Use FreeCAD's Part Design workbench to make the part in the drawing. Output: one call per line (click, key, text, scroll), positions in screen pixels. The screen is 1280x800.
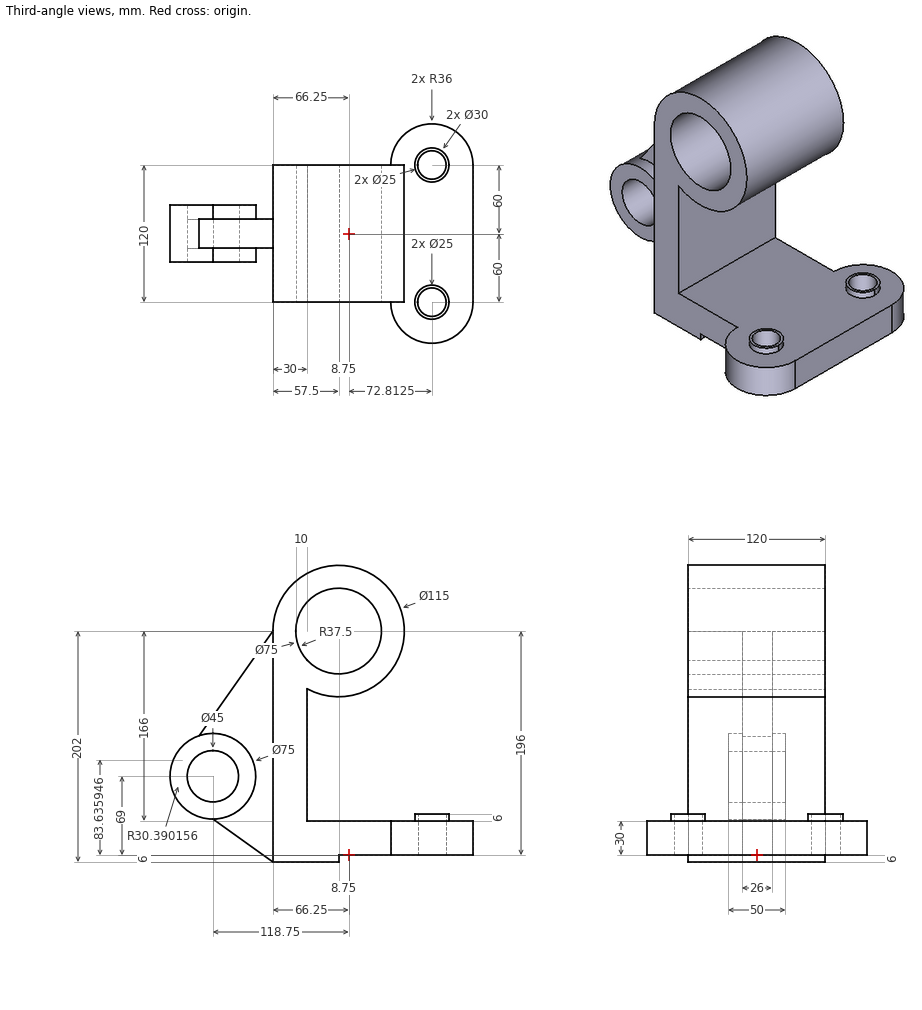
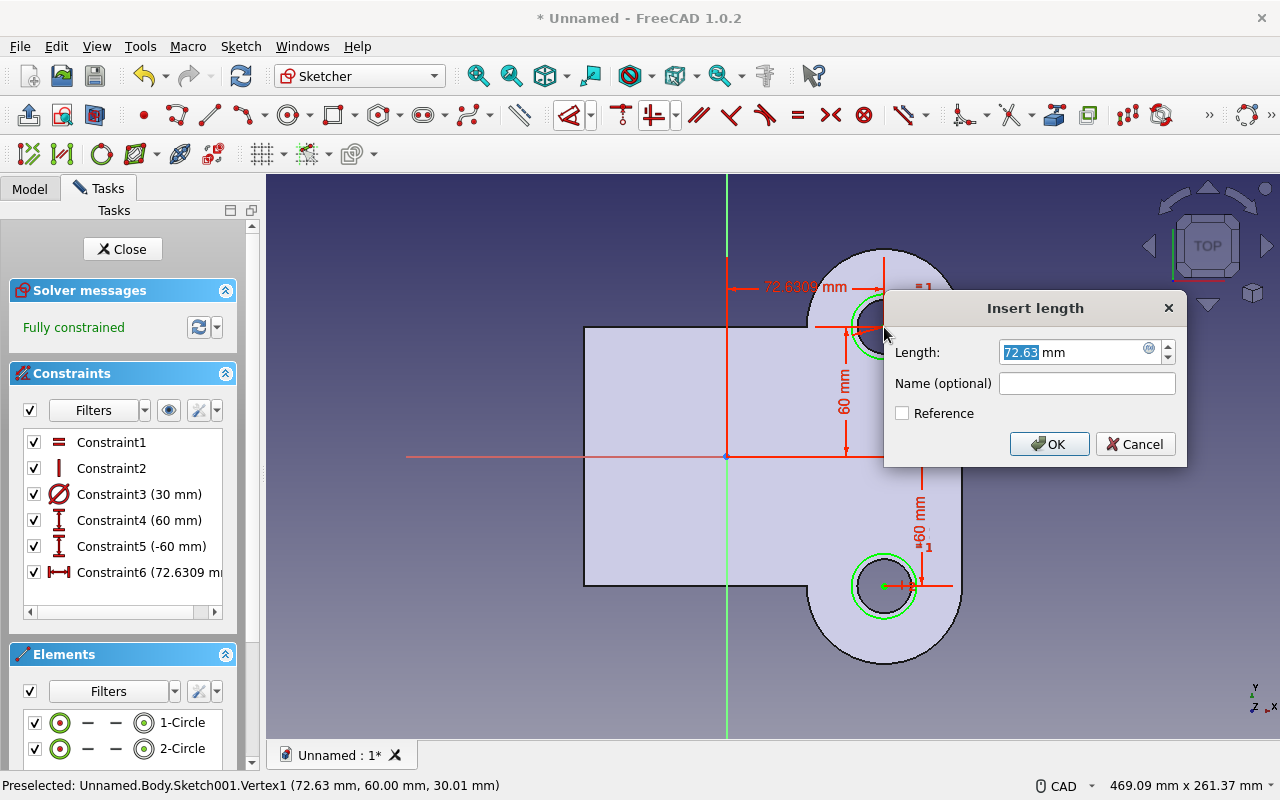
text(72.8125)
key(Return)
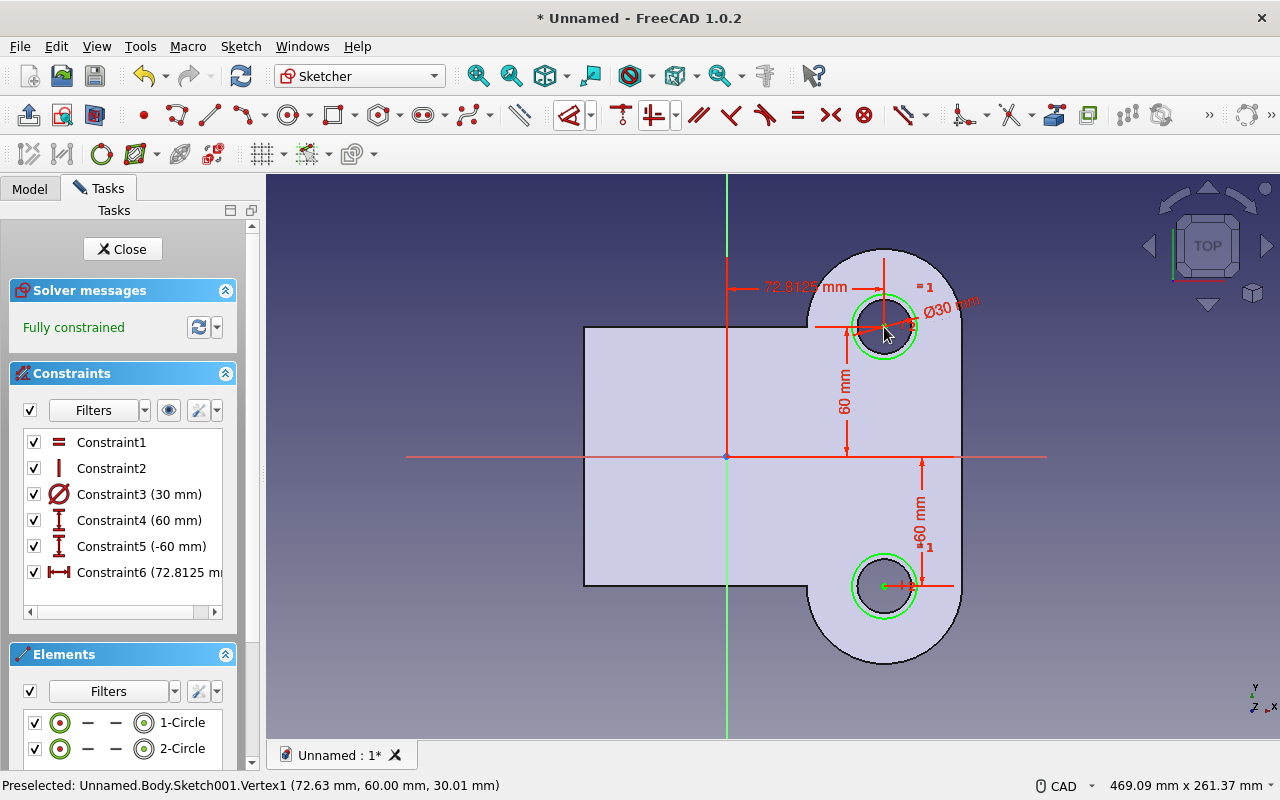
click(123, 249)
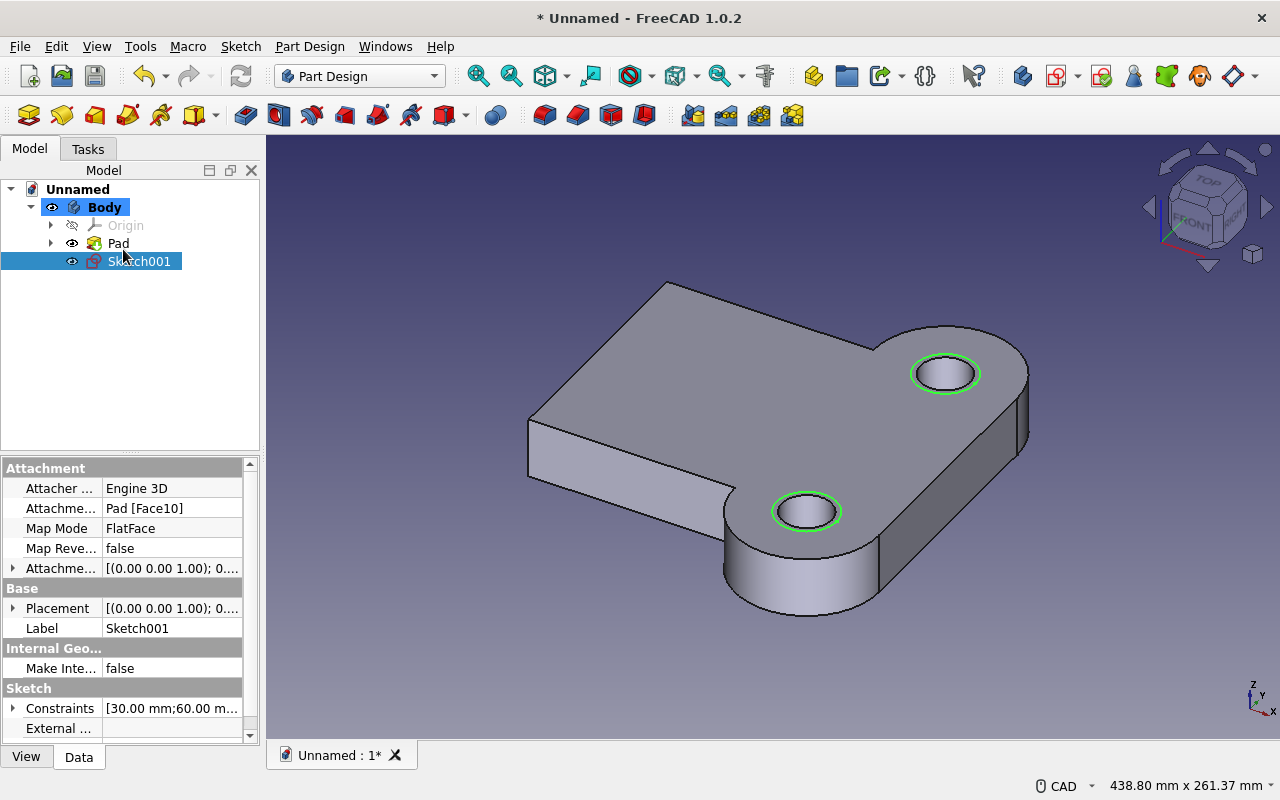
click(29, 116)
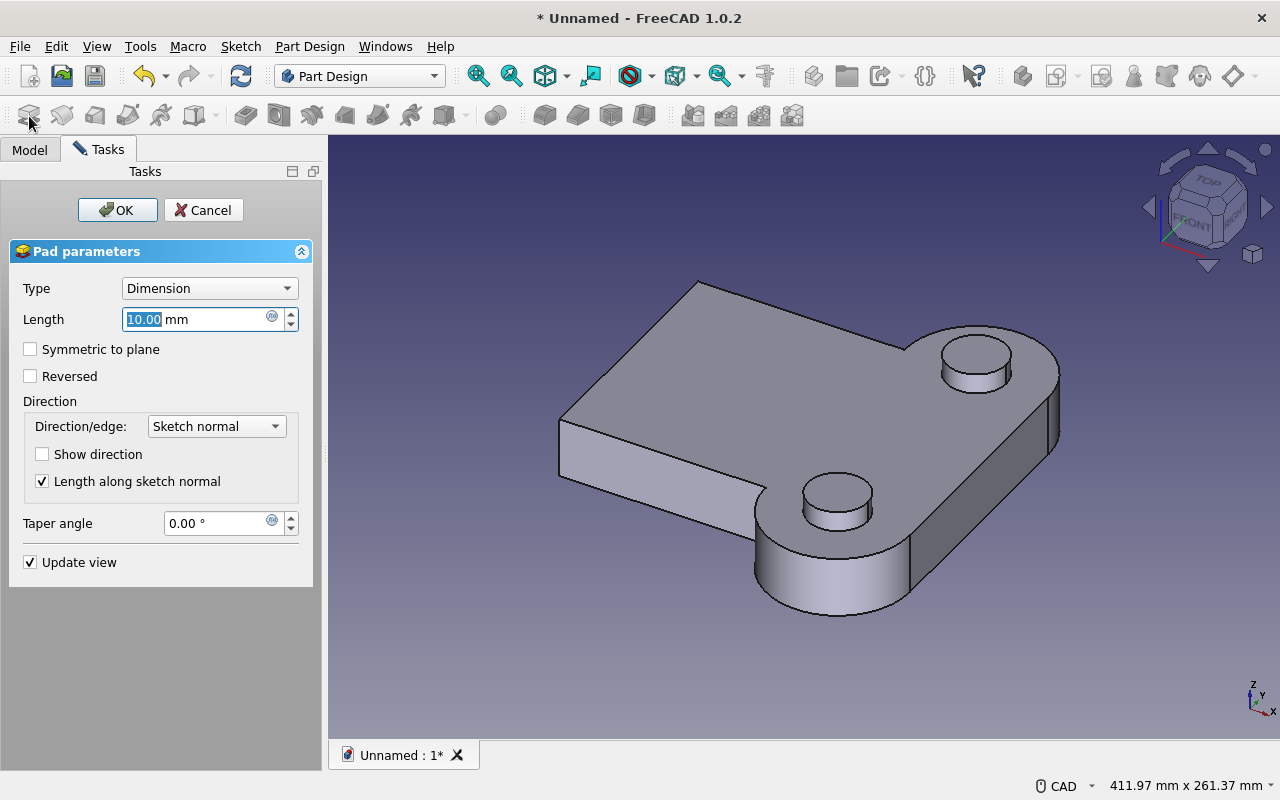
text(6)
key(Tab)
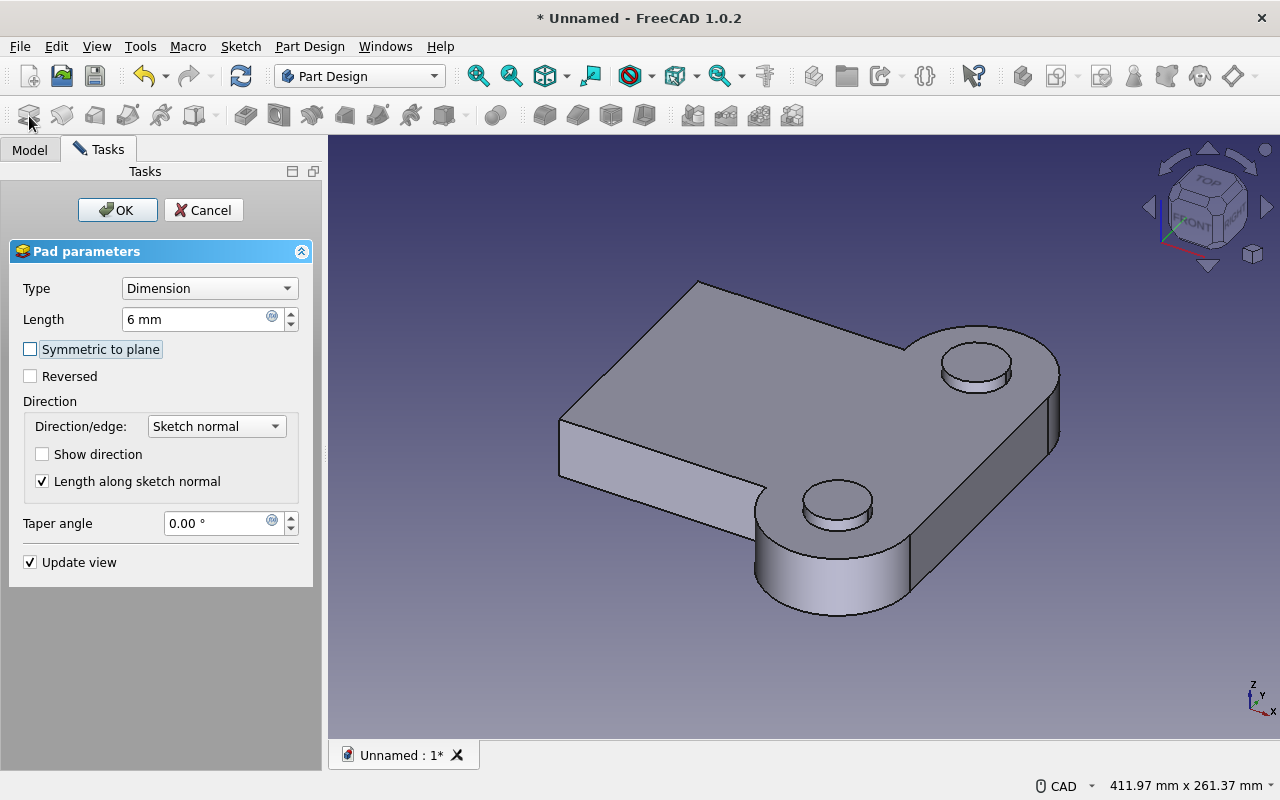
click(118, 210)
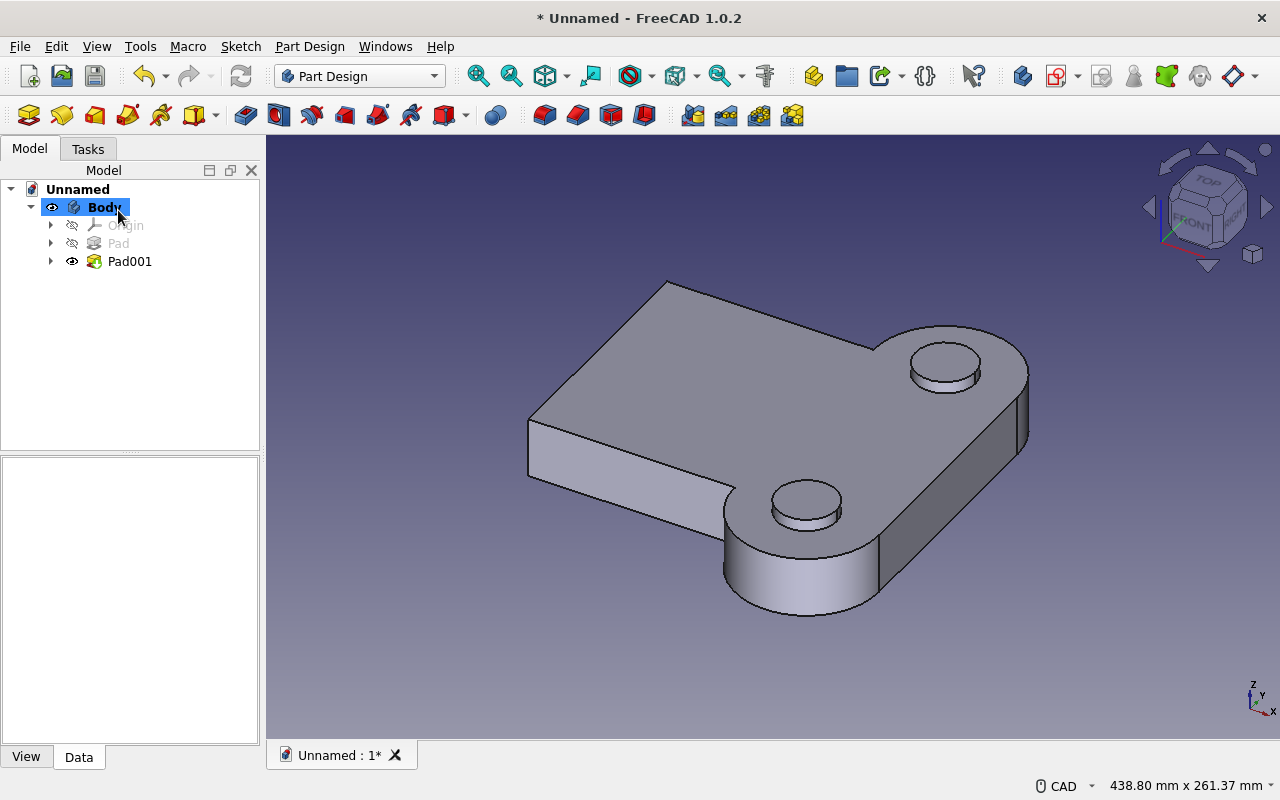
key(5)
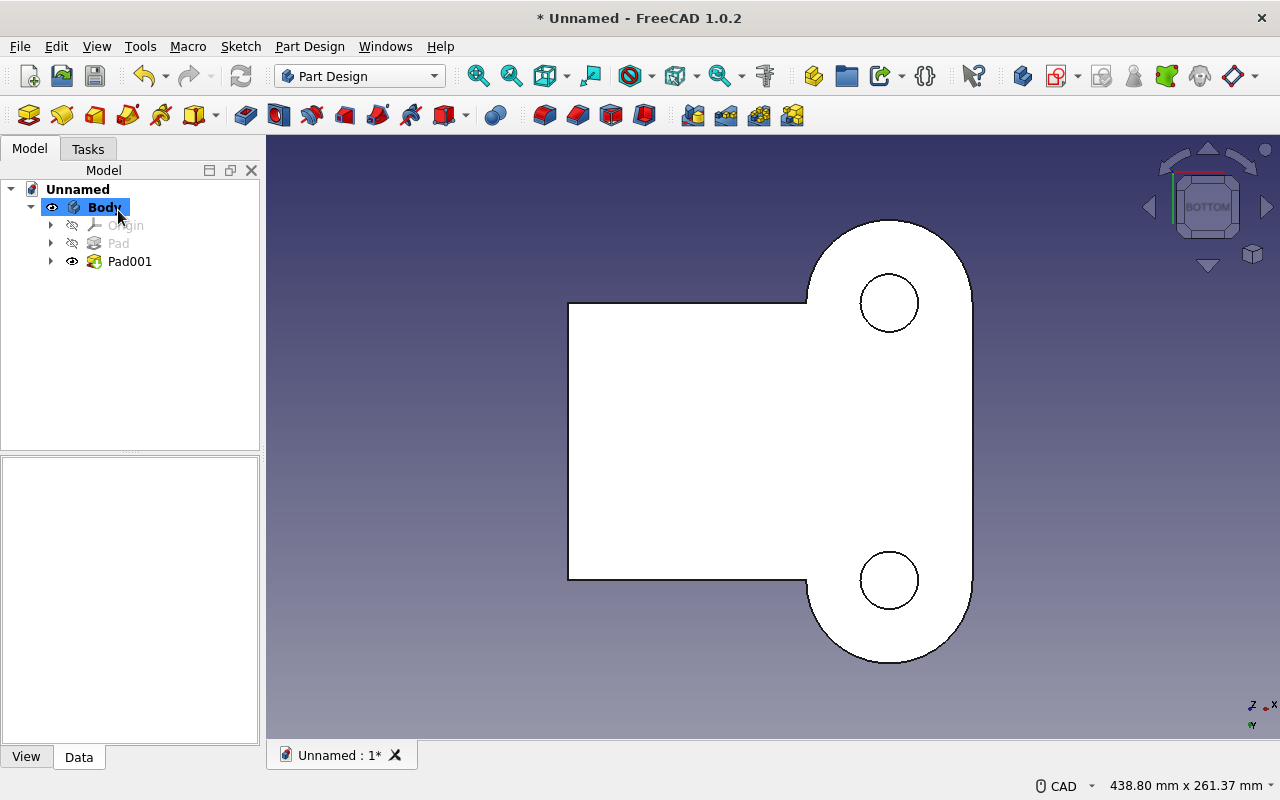
click(770, 441)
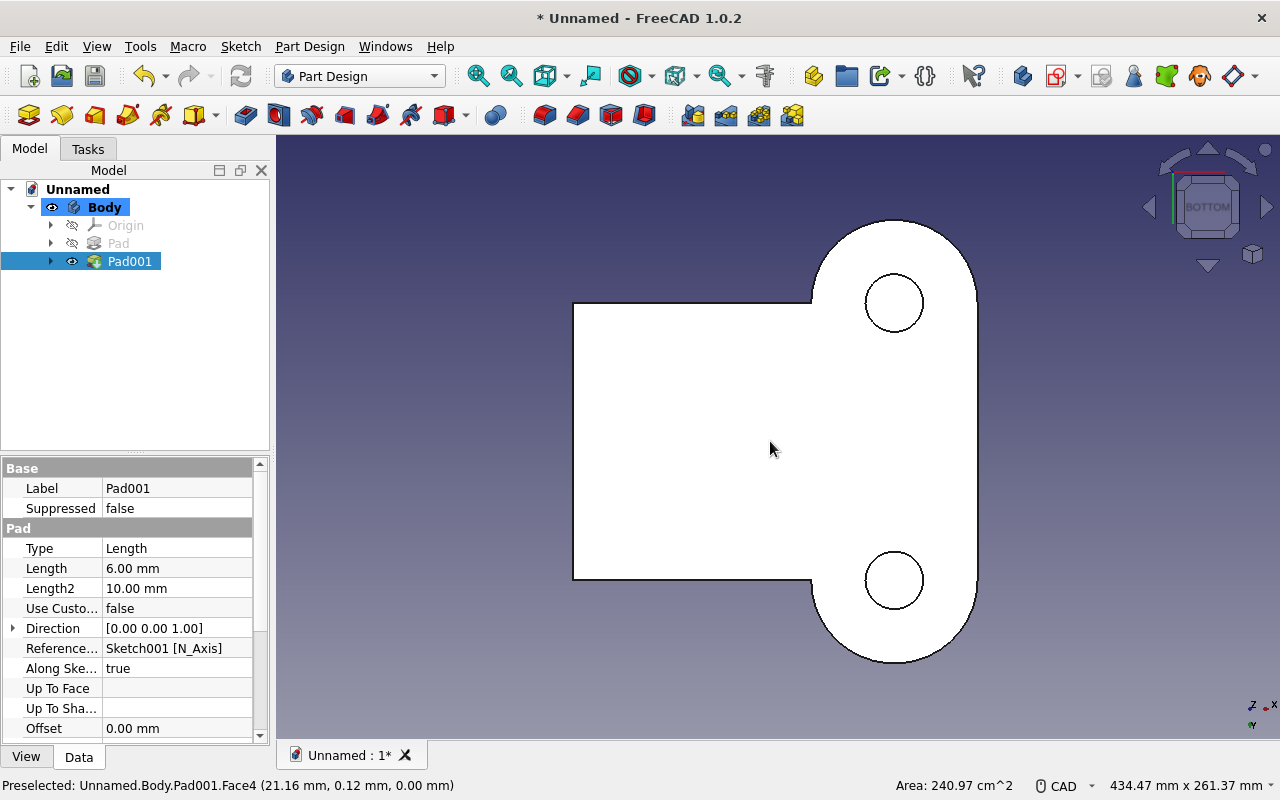
click(1056, 76)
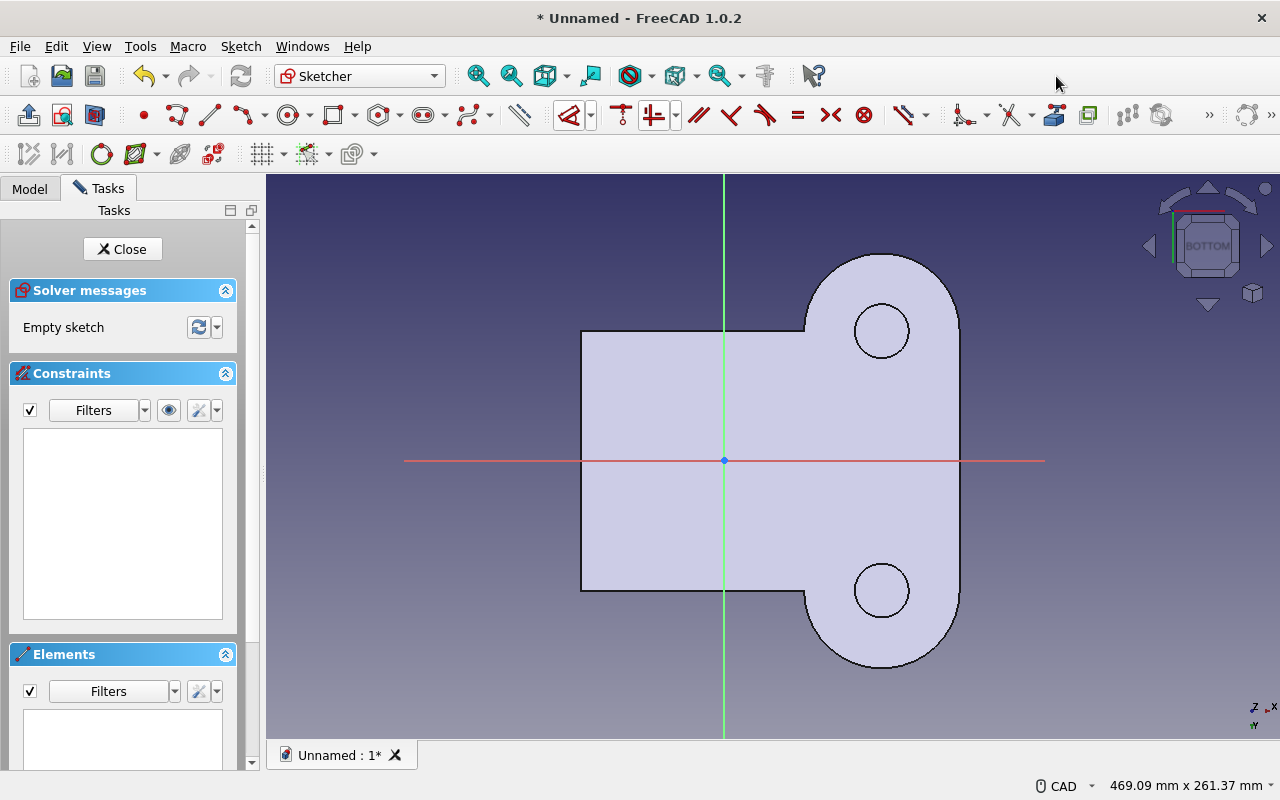
key(g)
key(c)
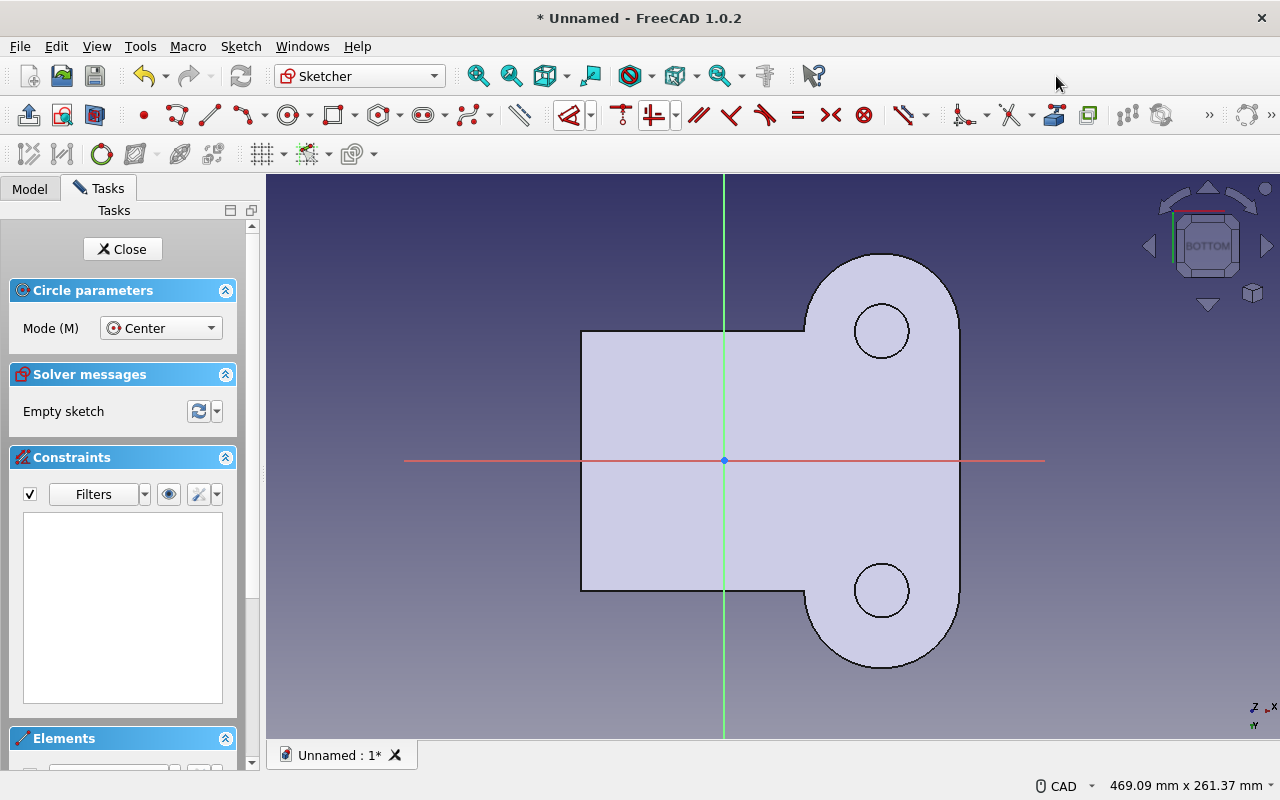
click(882, 591)
click(901, 572)